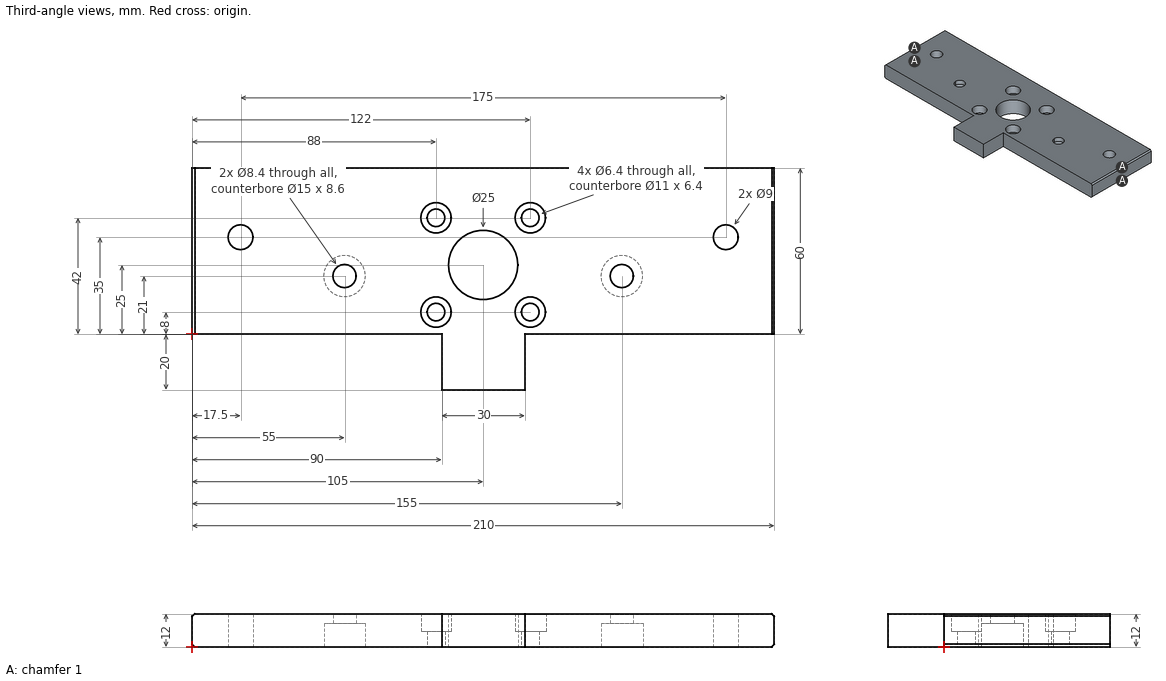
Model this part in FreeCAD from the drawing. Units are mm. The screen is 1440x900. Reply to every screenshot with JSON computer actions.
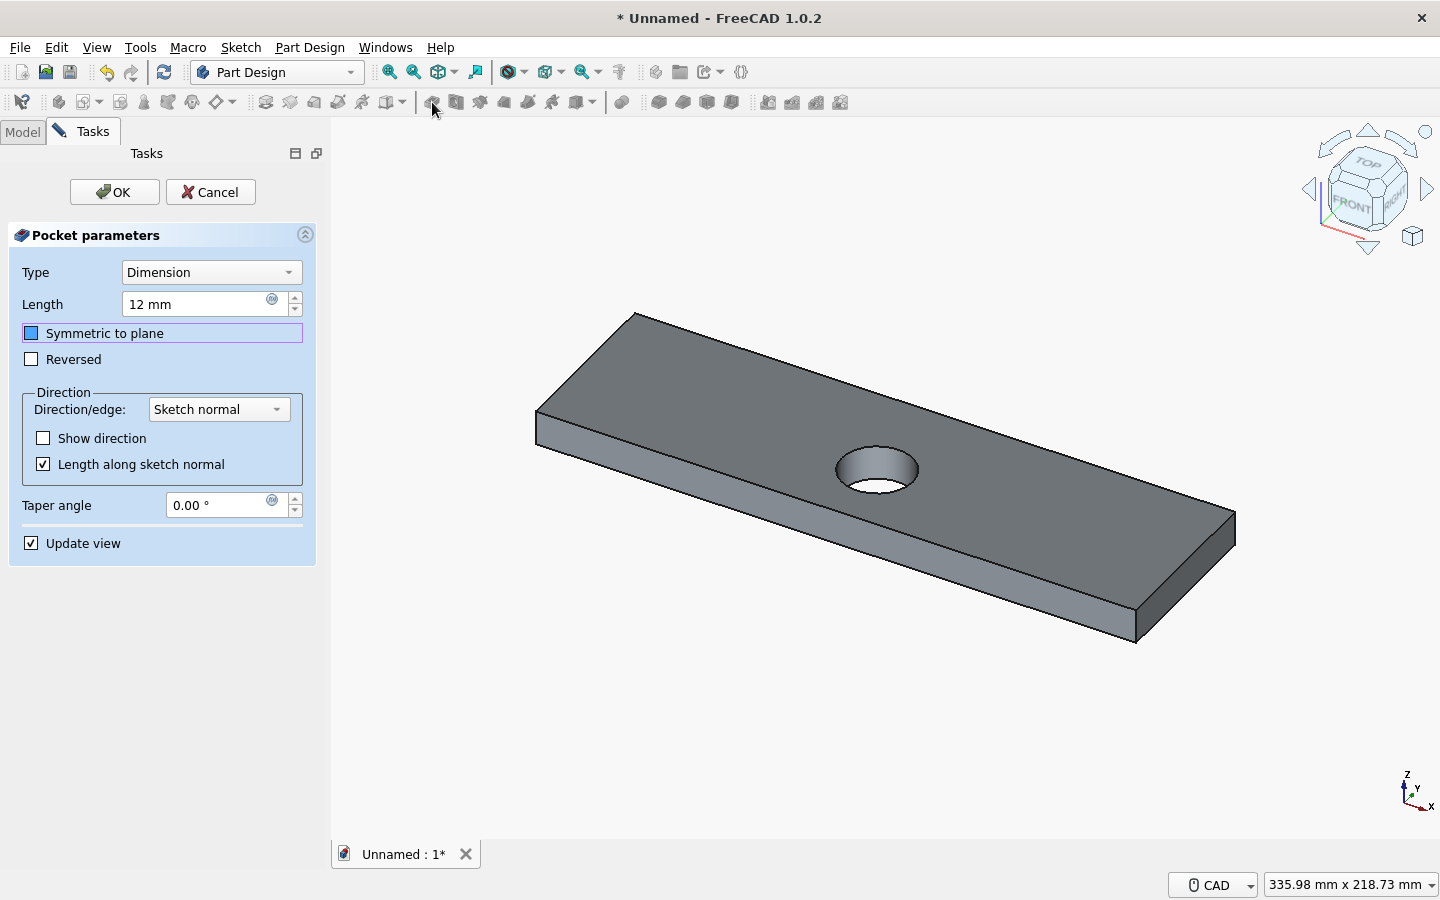
{"action": "left_click", "coordinate": [115, 192]}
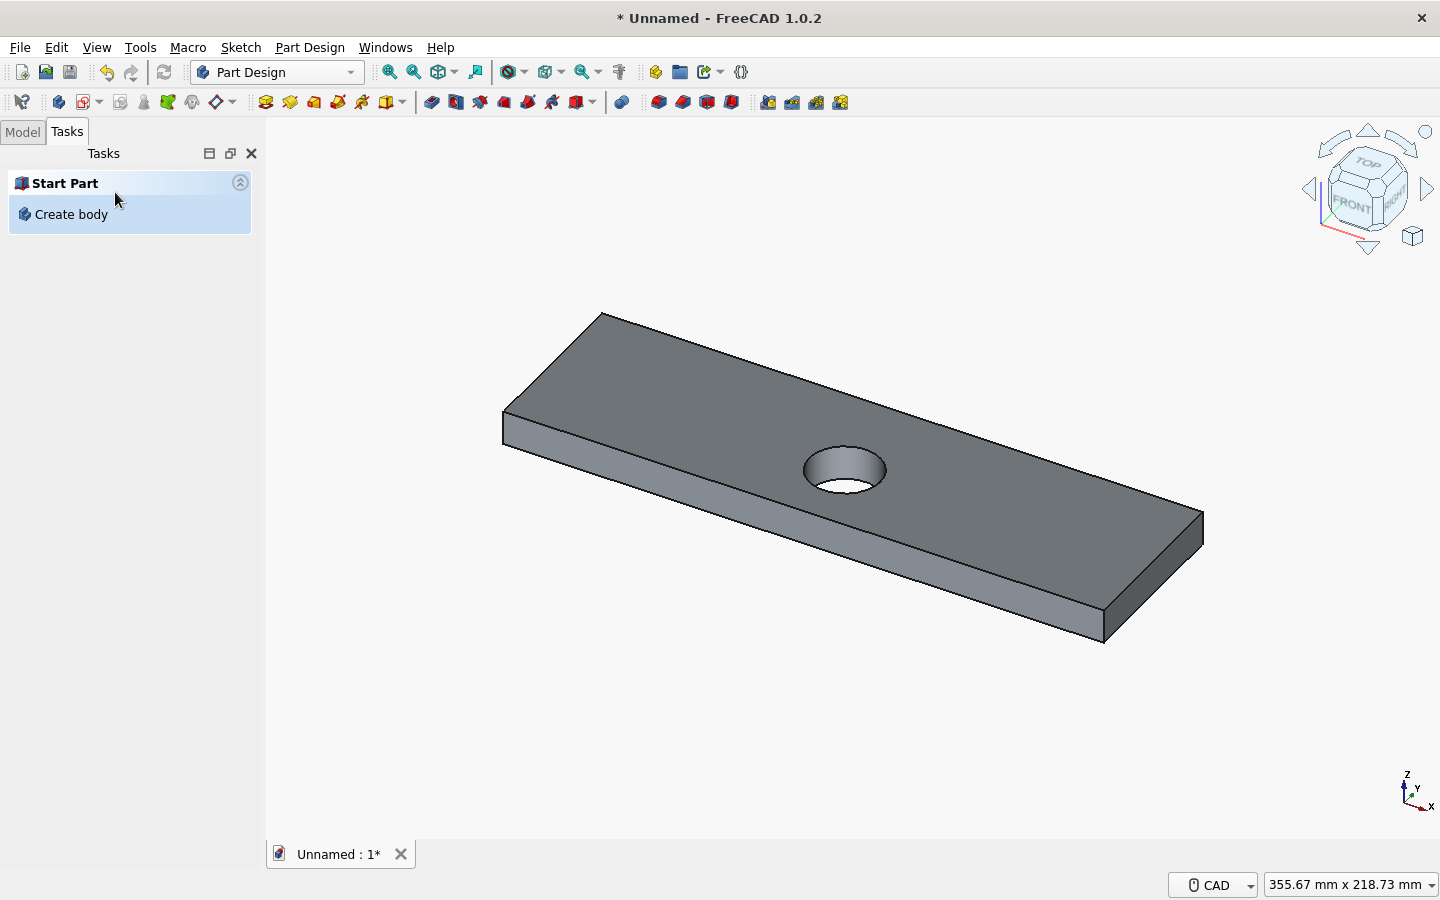
{"action": "left_click", "coordinate": [84, 102]}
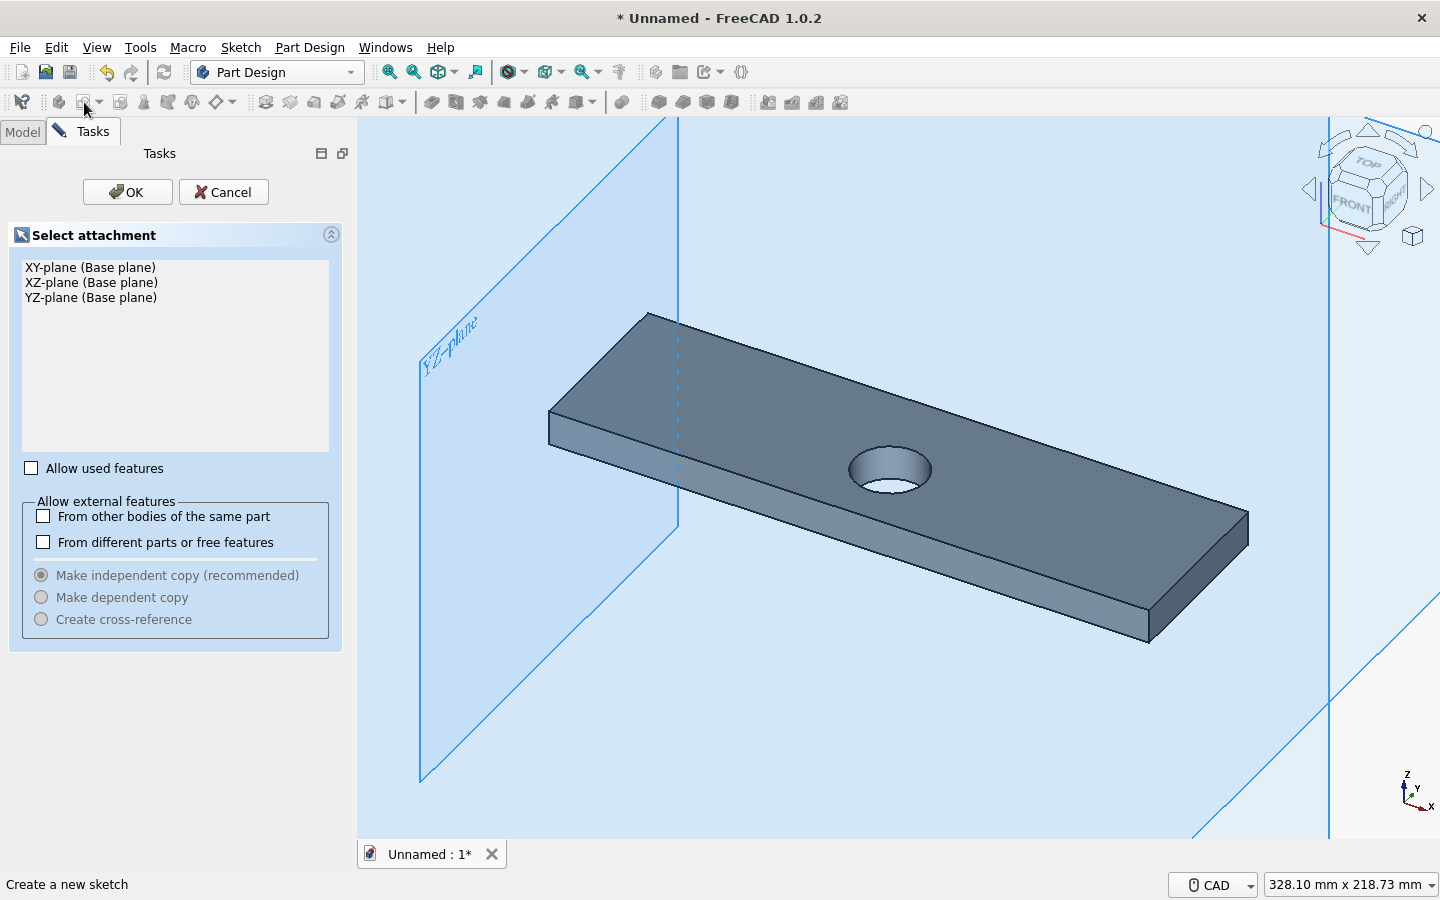
{"action": "left_click", "coordinate": [82, 268]}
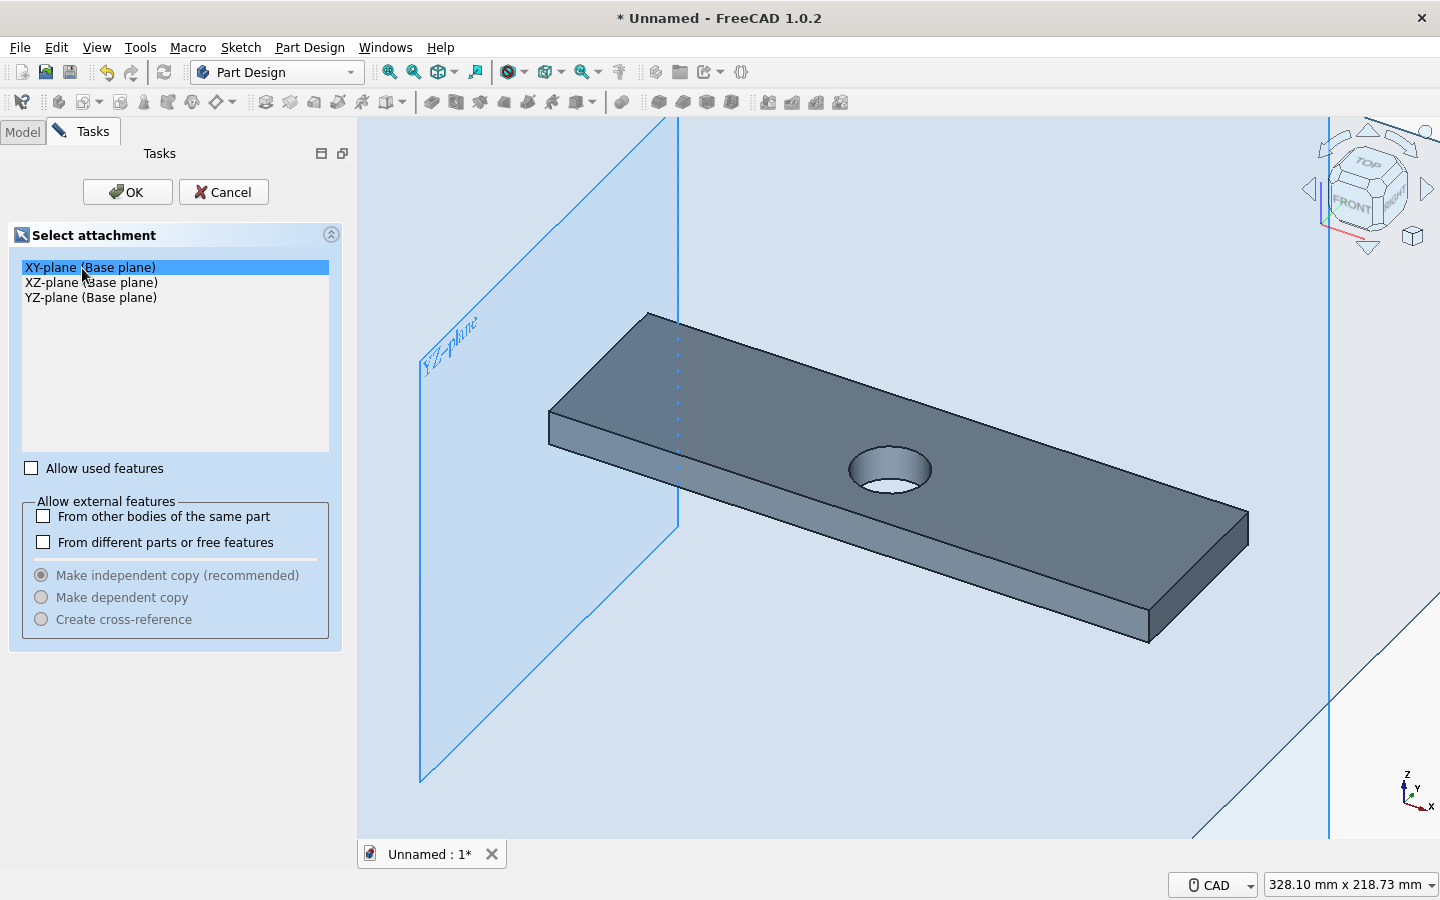
{"action": "left_click", "coordinate": [128, 192]}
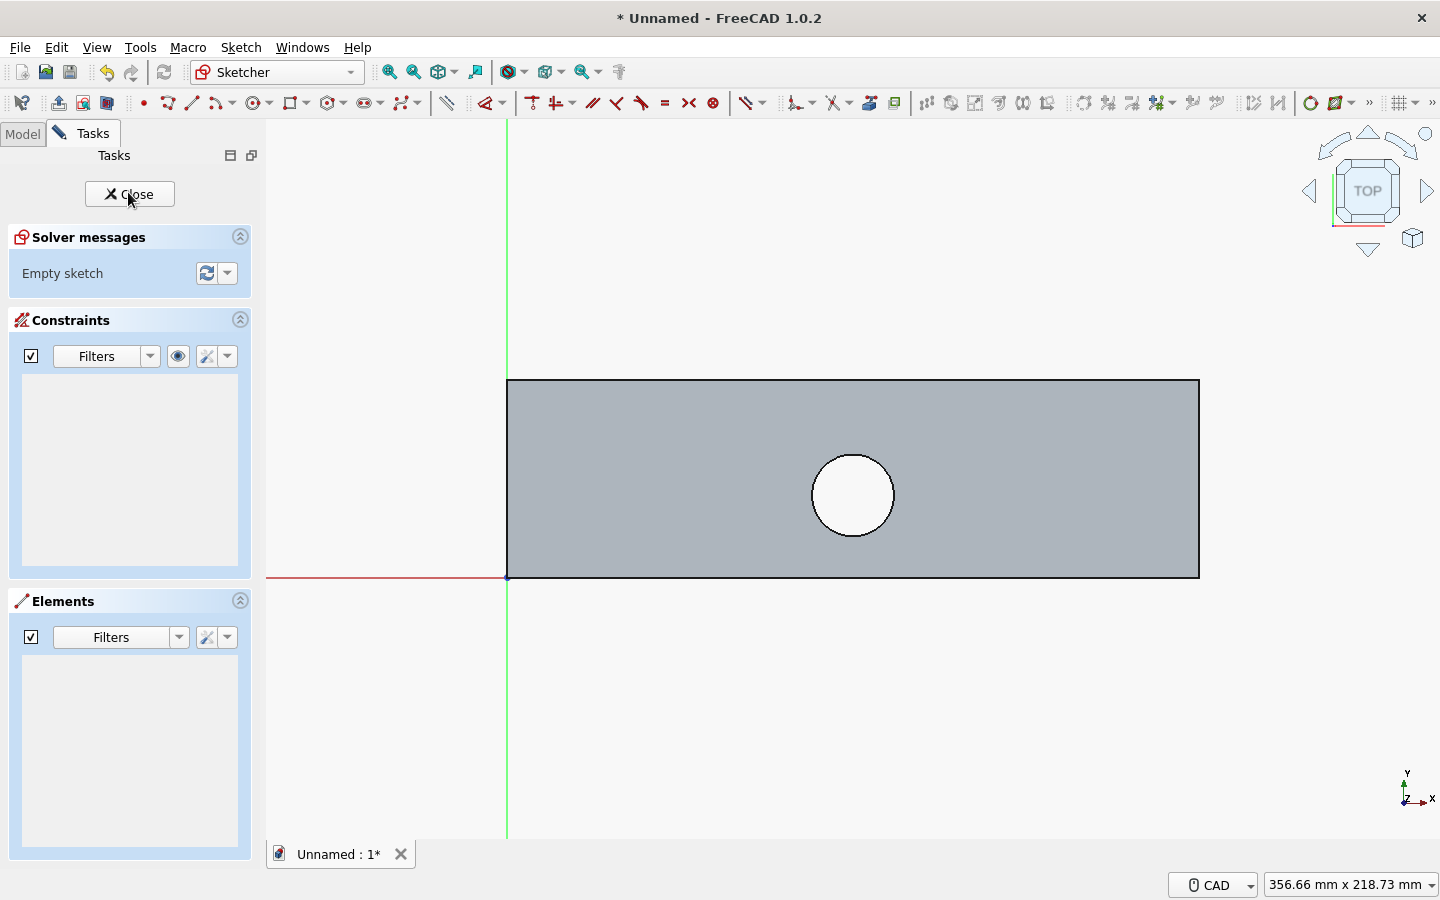
{"action": "key", "text": "q s"}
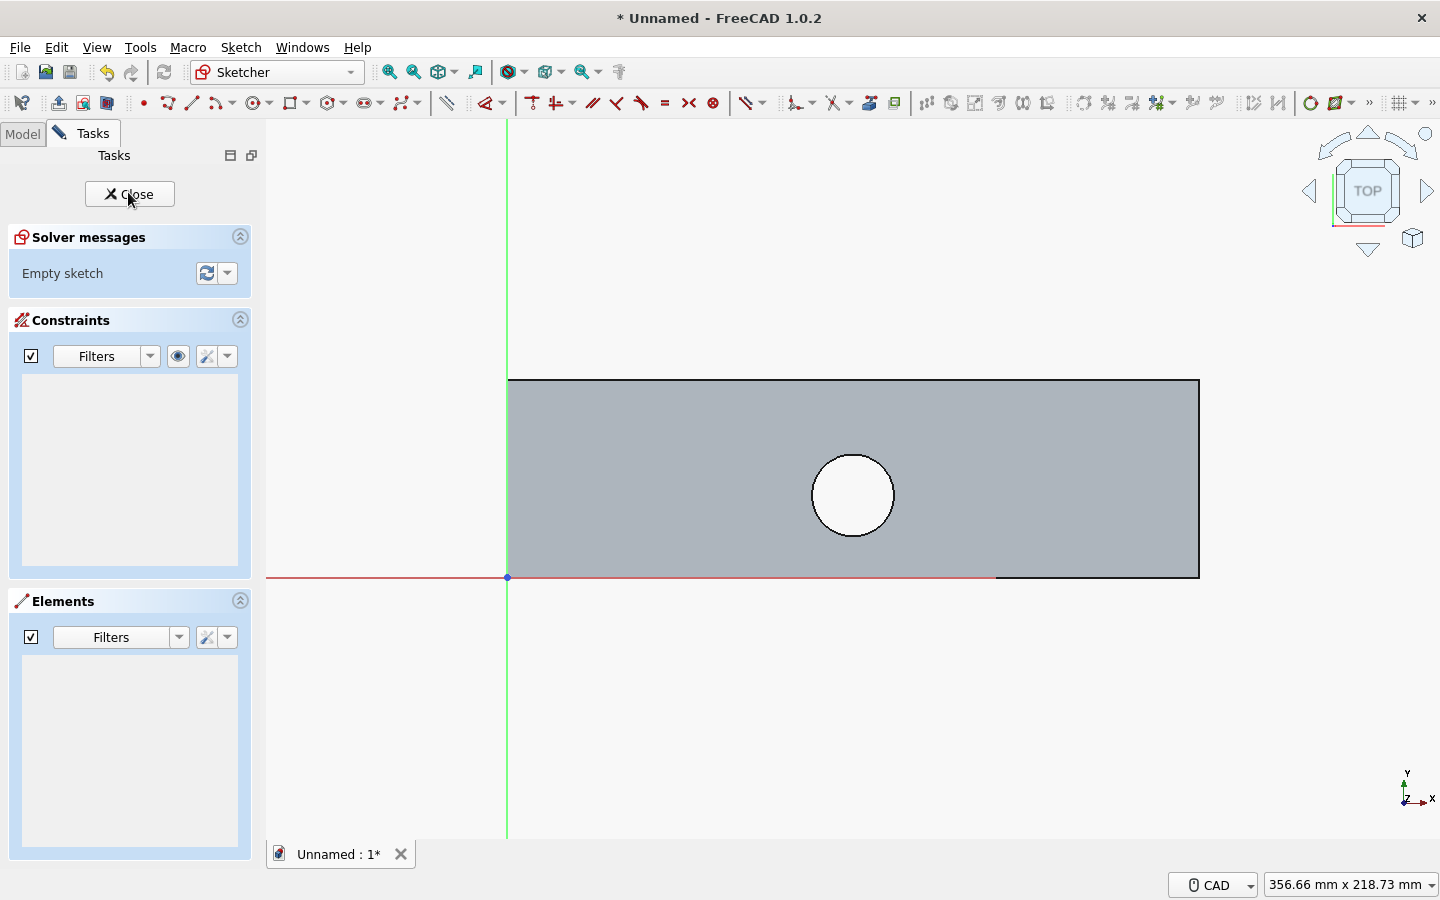
{"action": "key", "text": "g c"}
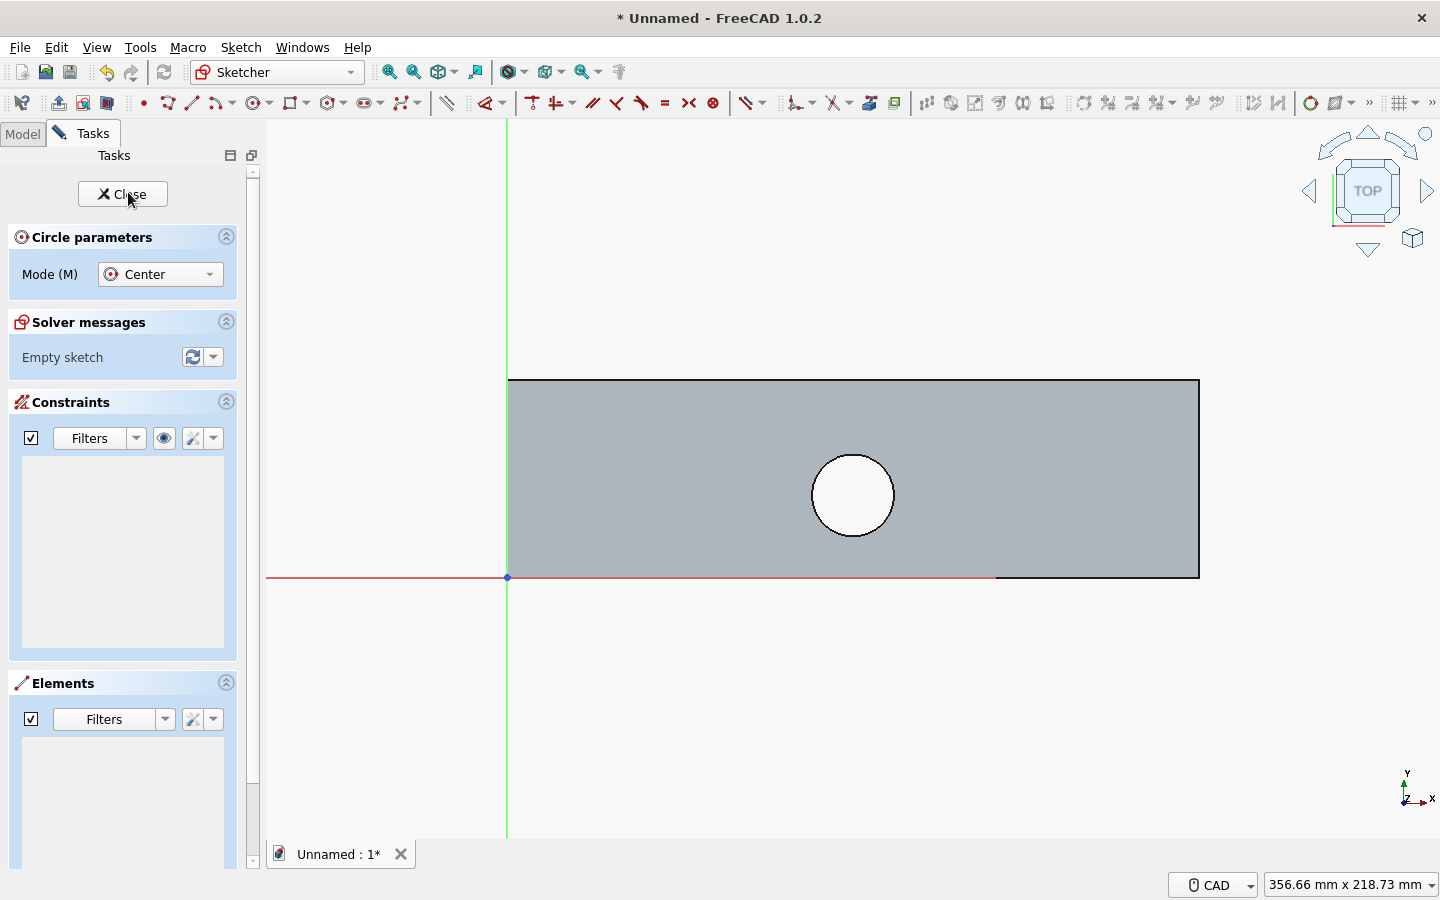
{"action": "scroll", "coordinate": [688, 509], "scroll_direction": "up", "scroll_amount": 3}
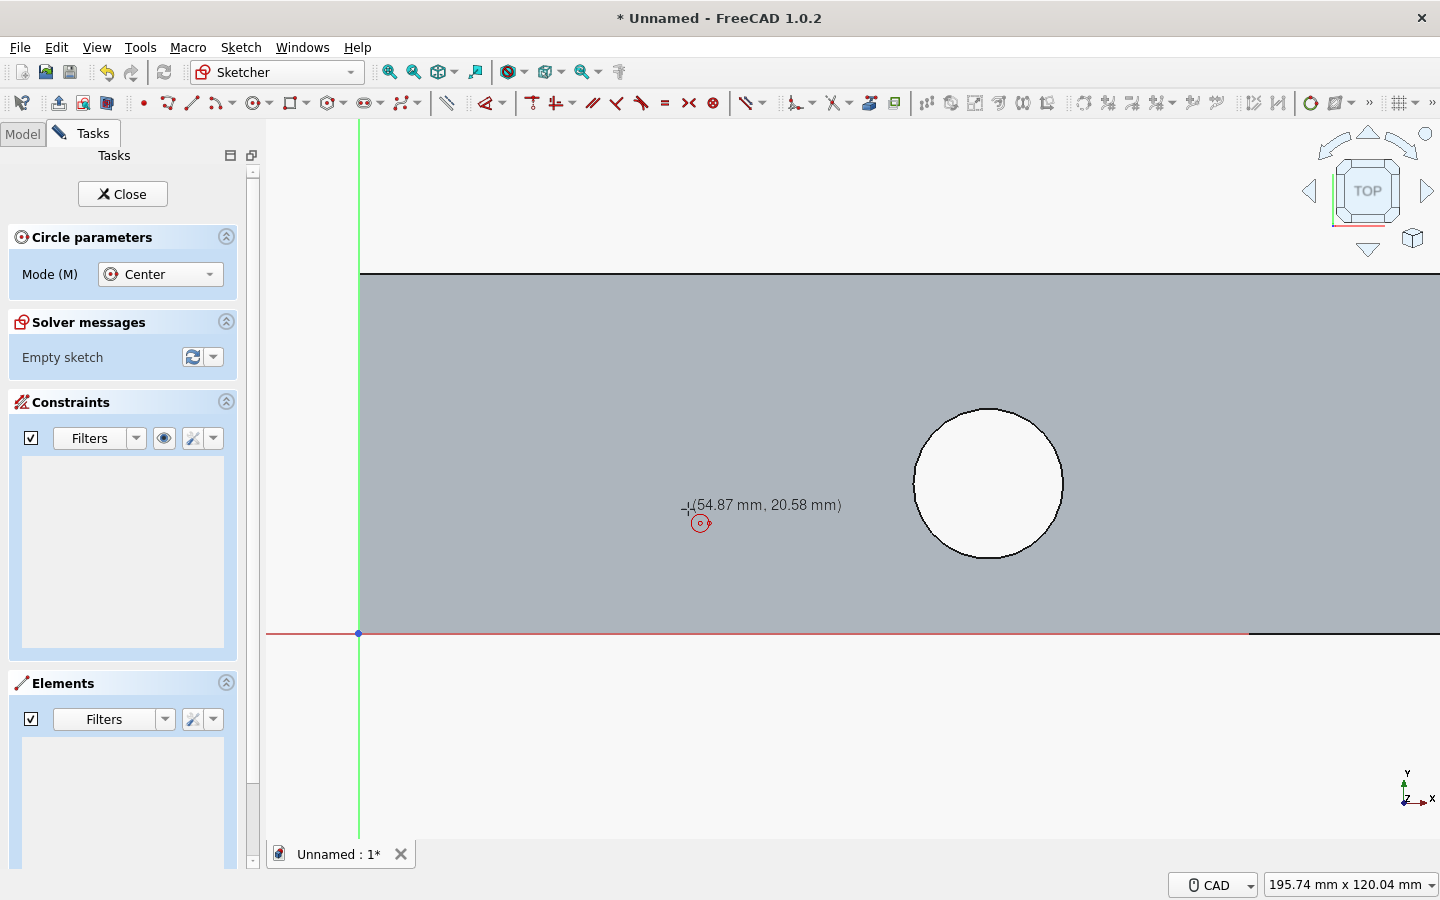
{"action": "left_click", "coordinate": [688, 508]}
{"action": "left_click", "coordinate": [706, 490]}